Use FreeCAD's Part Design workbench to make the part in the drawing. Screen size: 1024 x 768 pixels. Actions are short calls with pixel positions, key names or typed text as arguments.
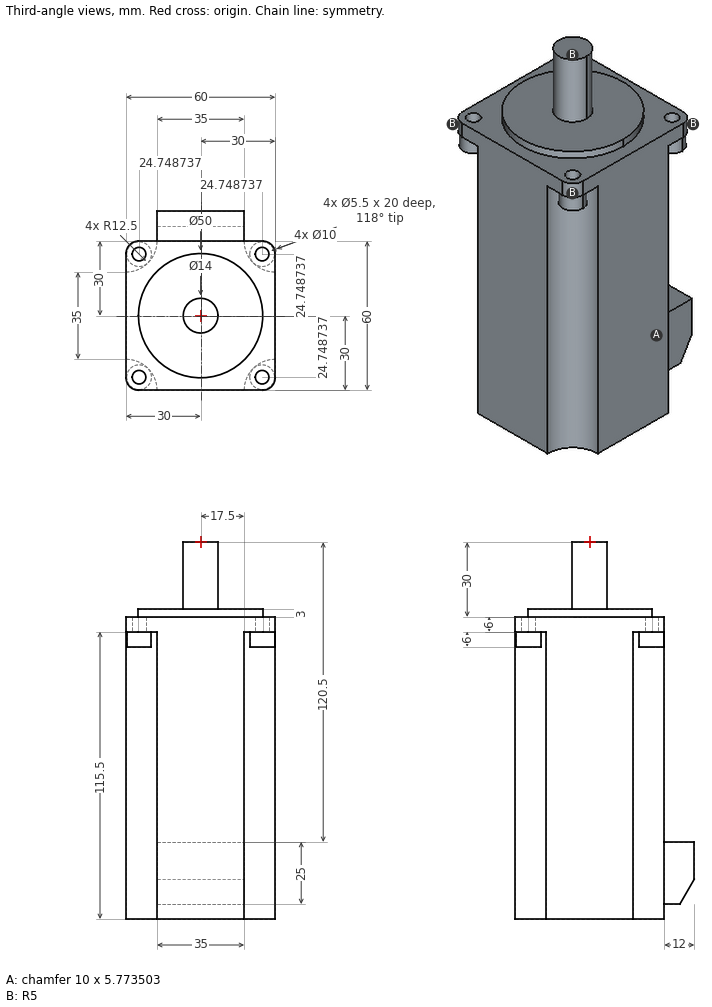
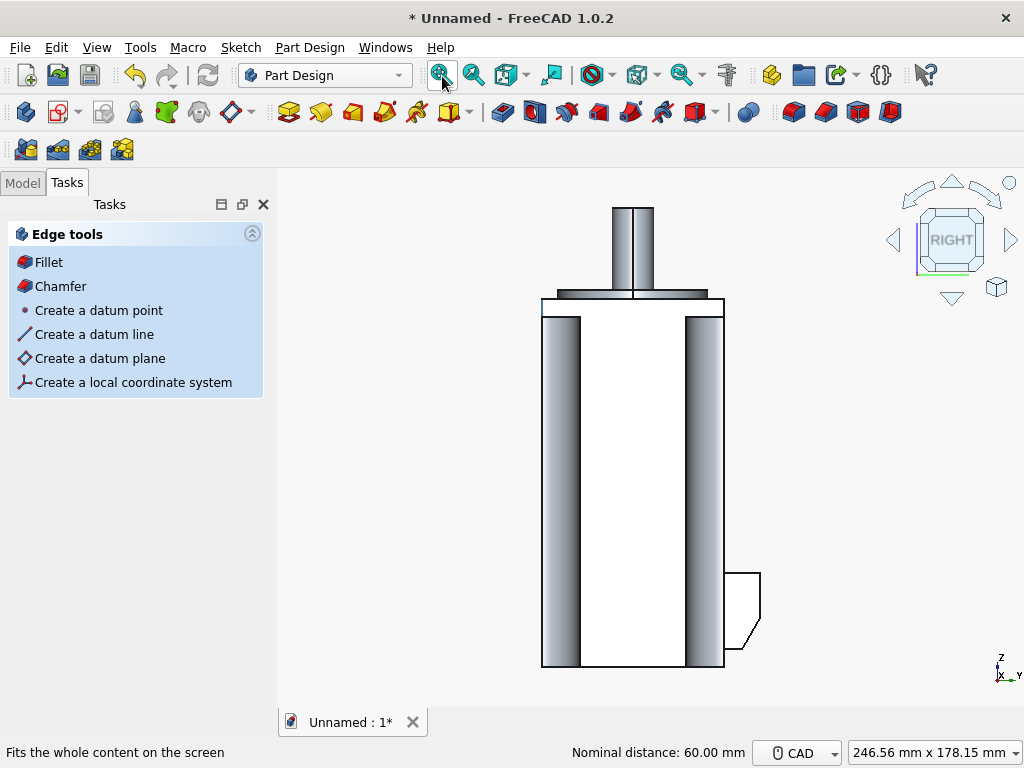
click(724, 307, ctrl)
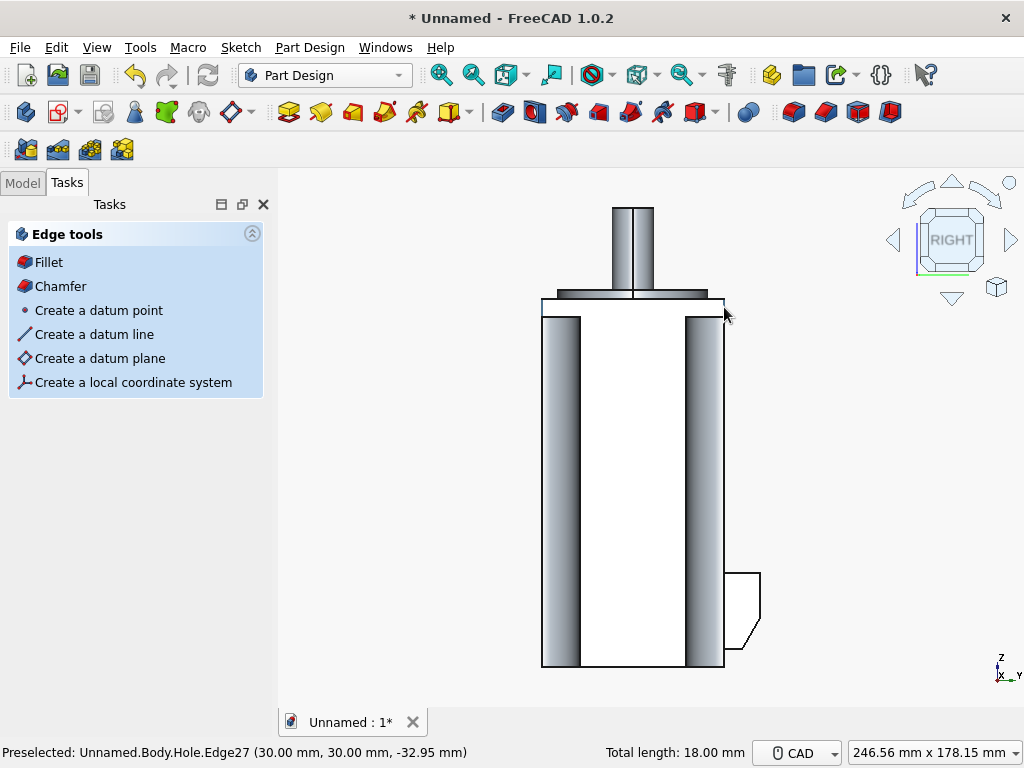
scroll(724, 307, up, 4)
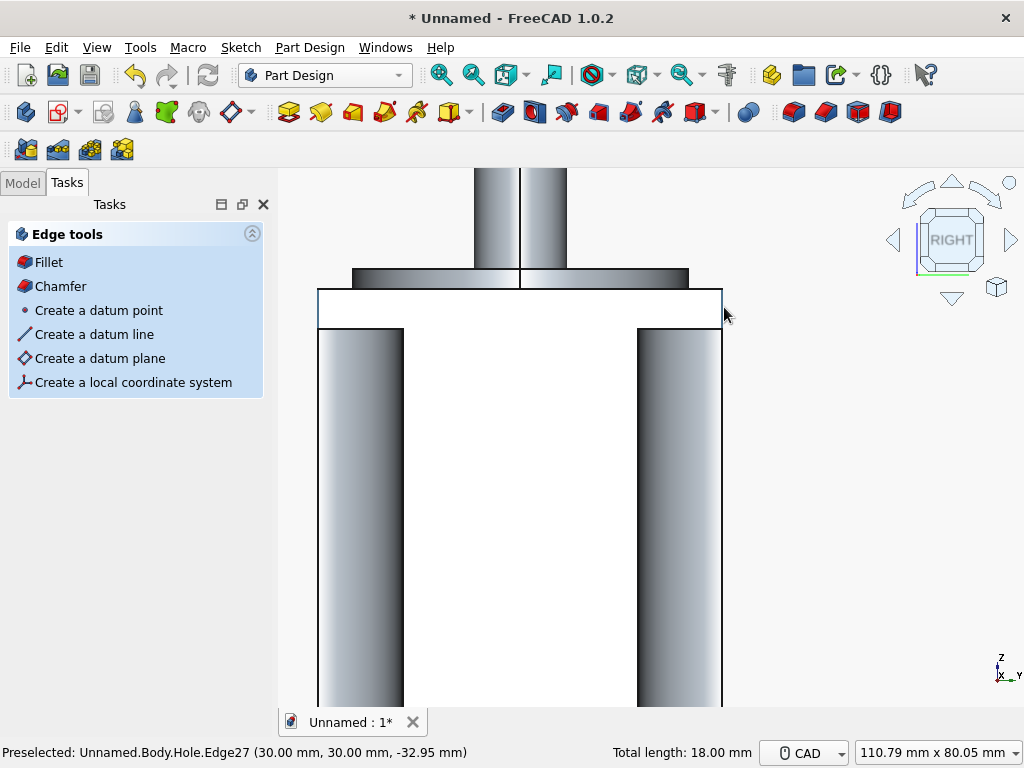
click(442, 76)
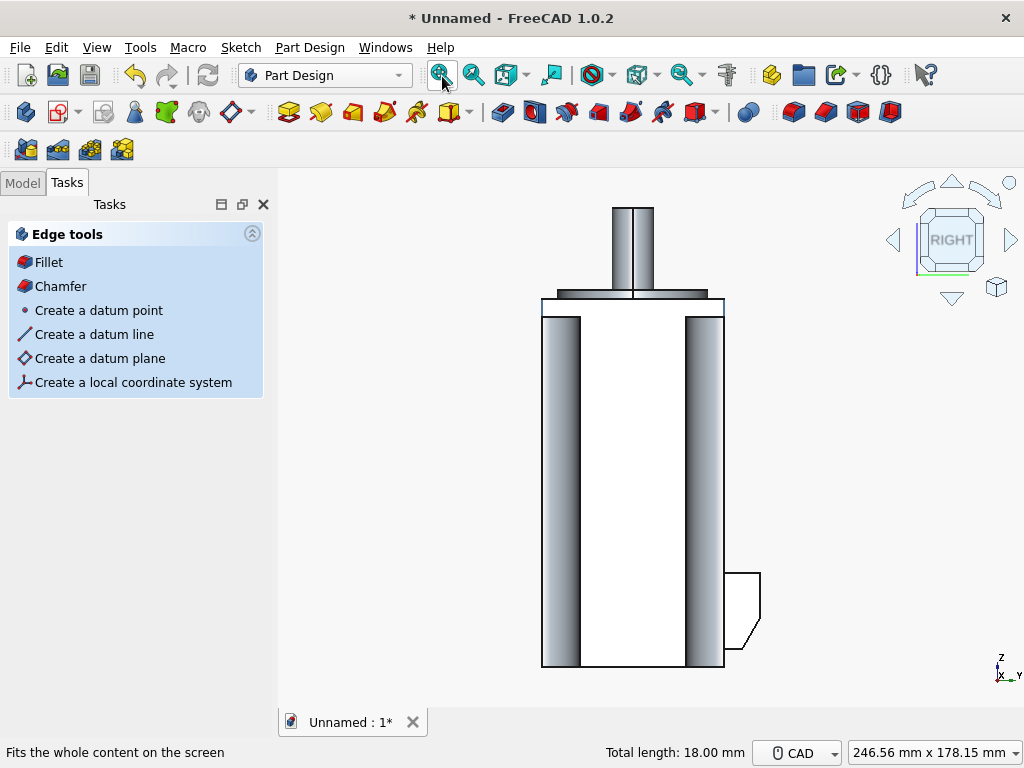
key(5)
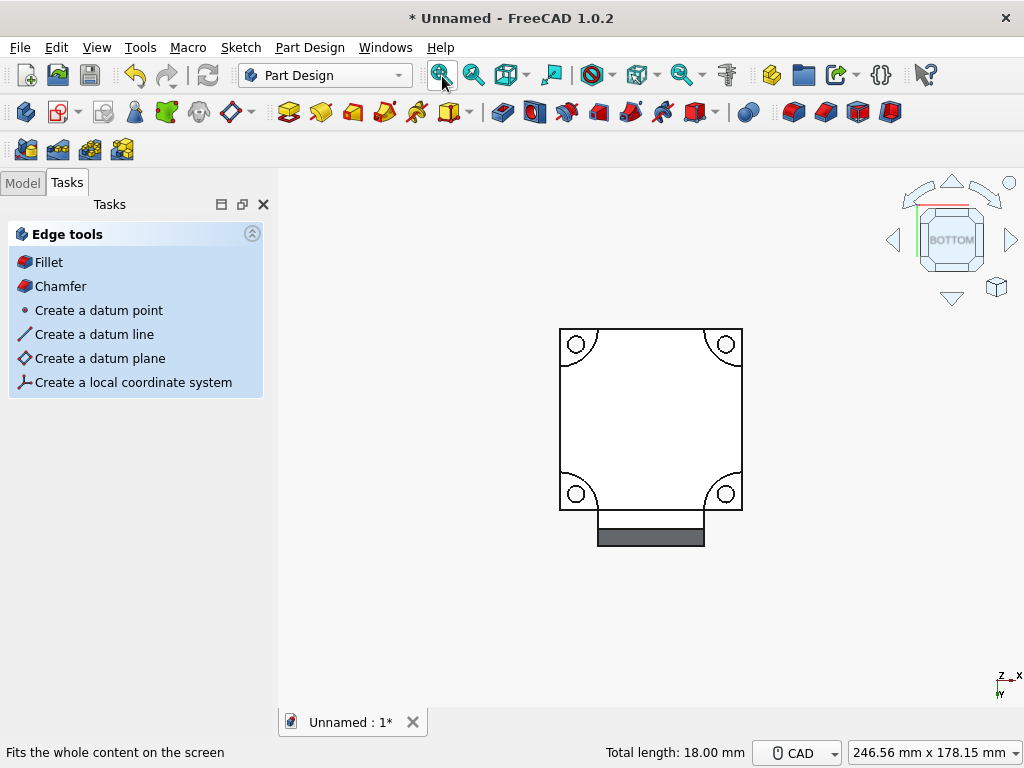
click(442, 76)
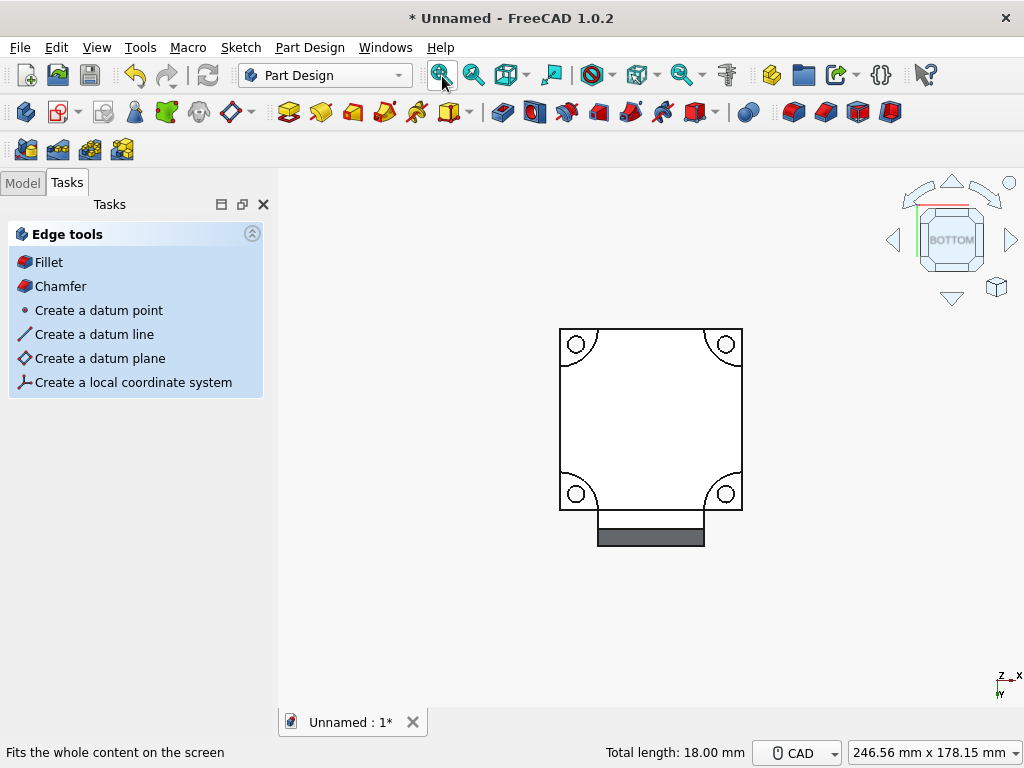
scroll(560, 509, up, 4)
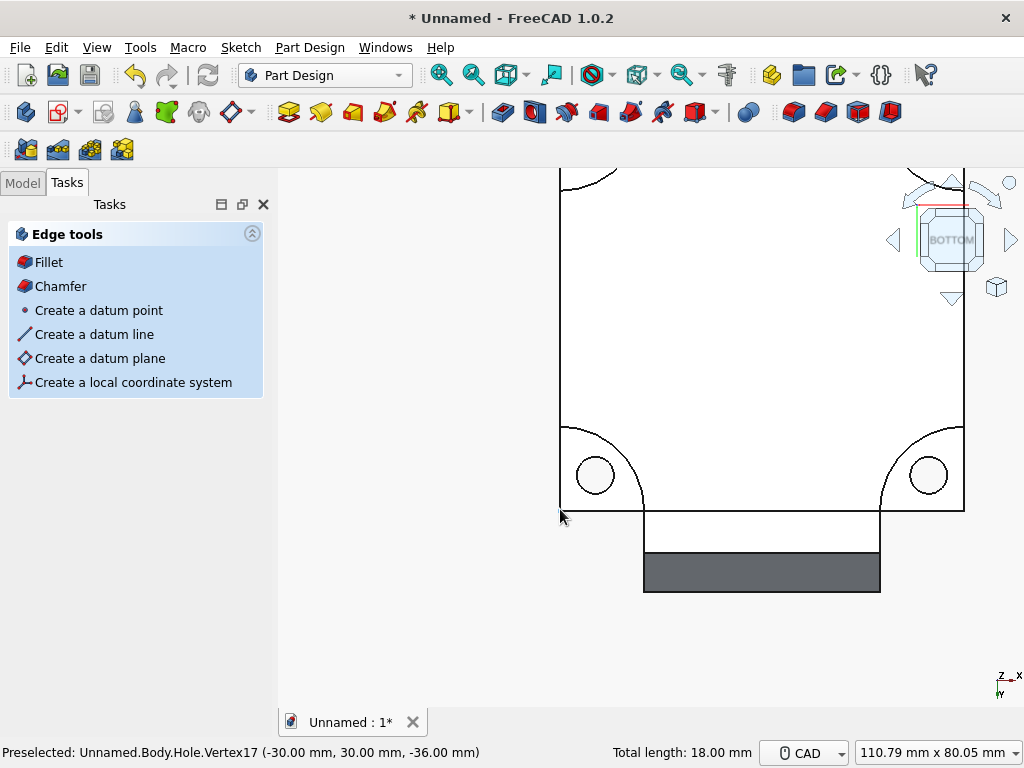
click(442, 76)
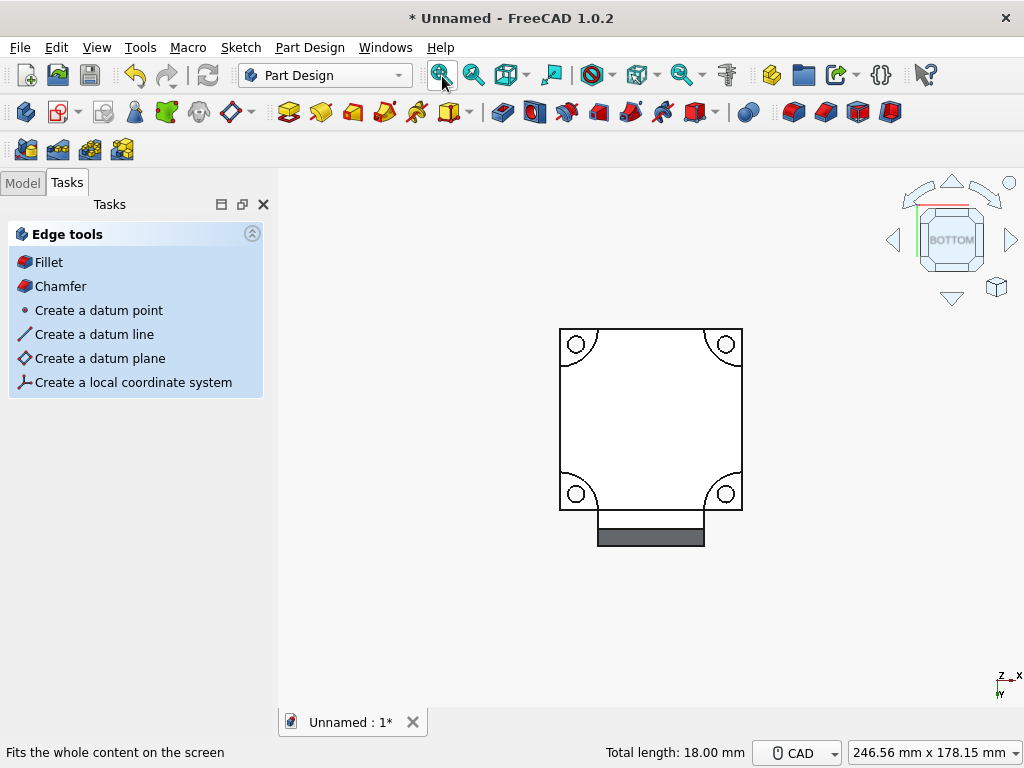
key(4)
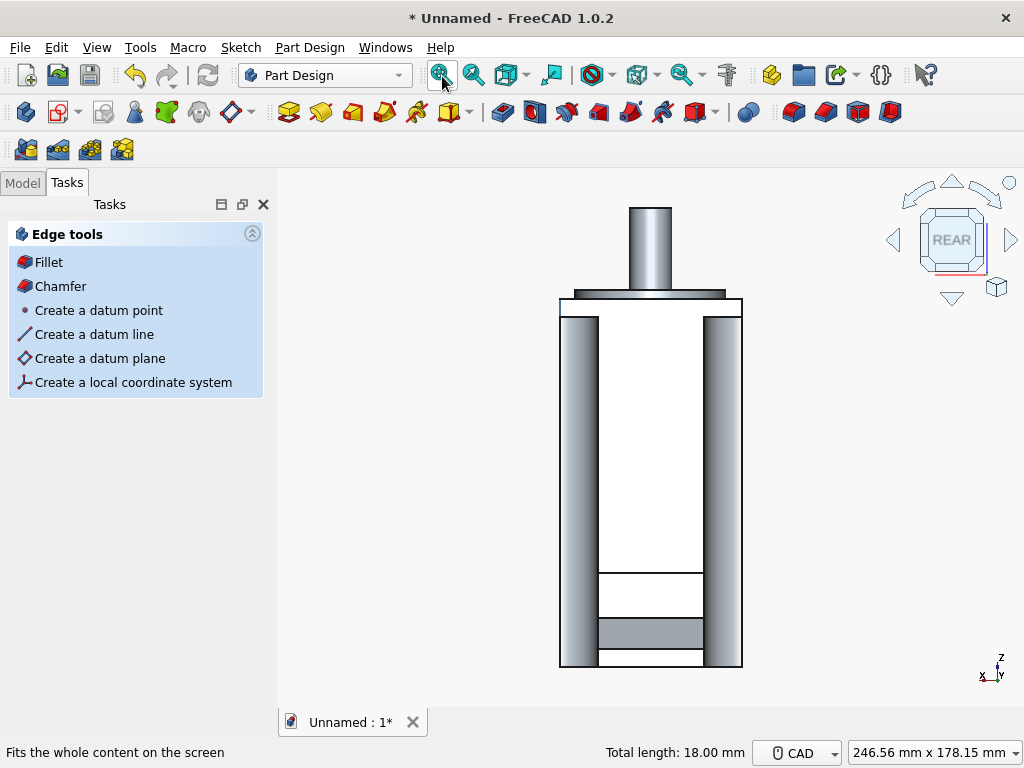
click(742, 307, ctrl)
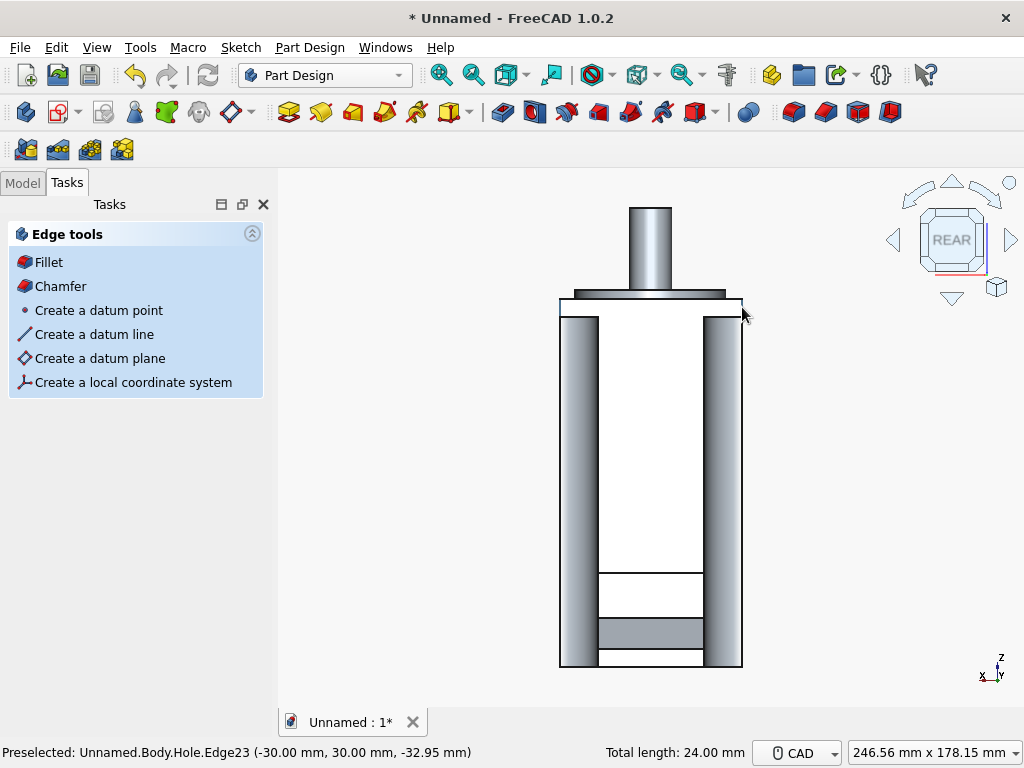
click(794, 112)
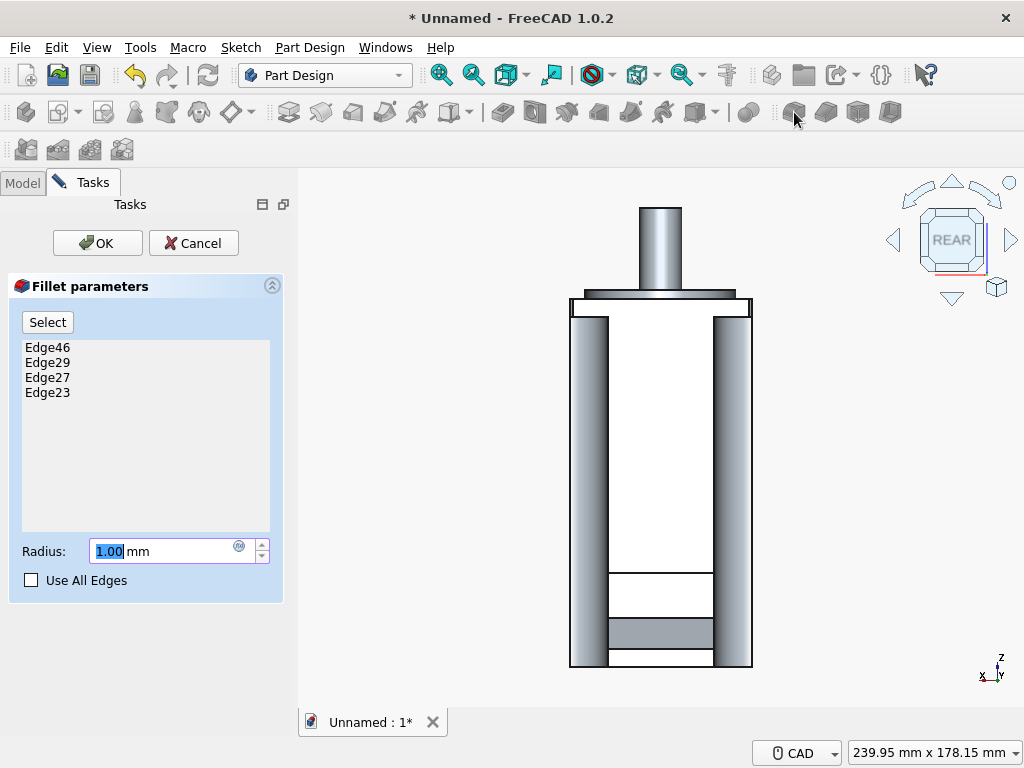
text(5)
key(Tab)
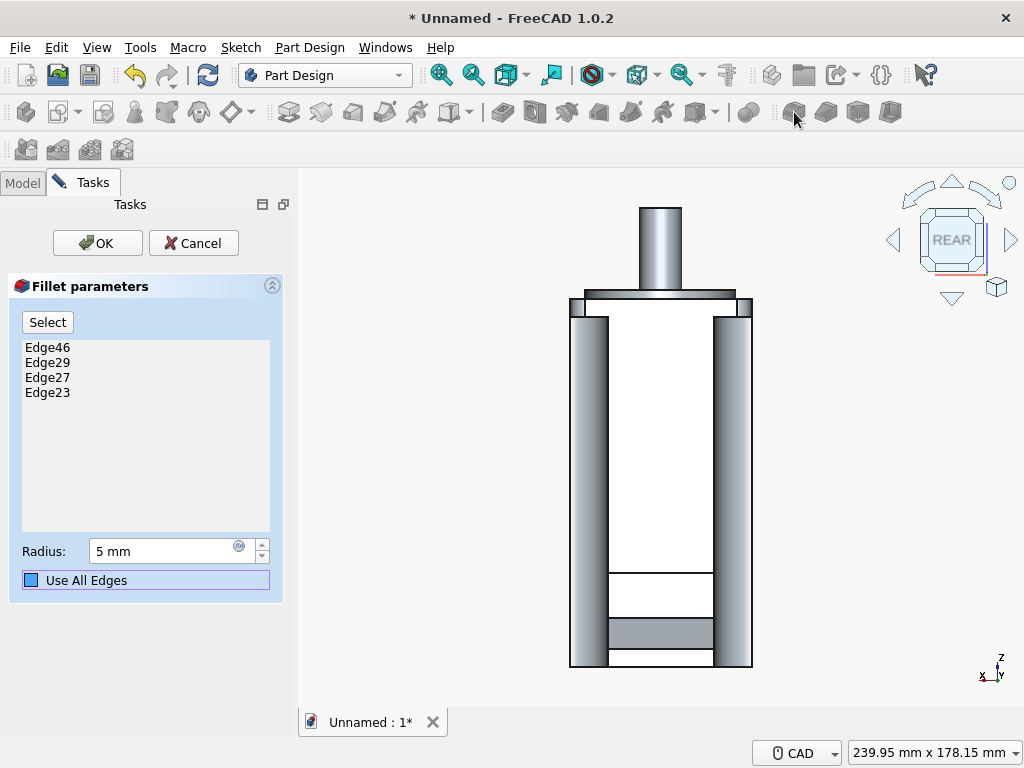
click(98, 243)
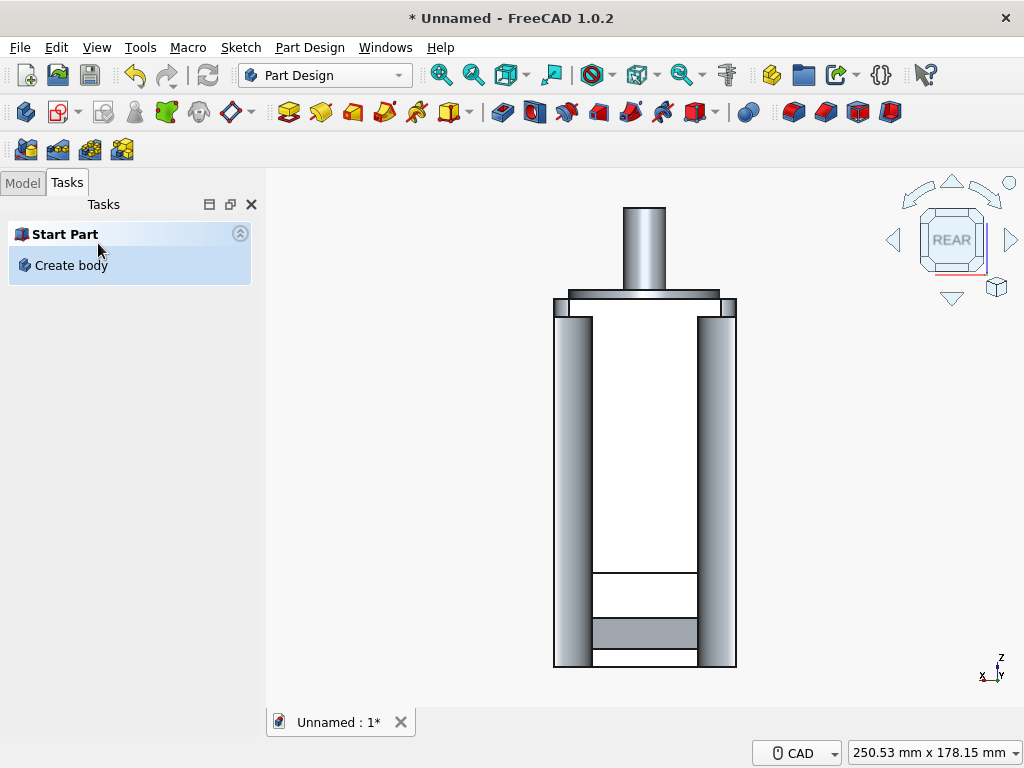
key(5)